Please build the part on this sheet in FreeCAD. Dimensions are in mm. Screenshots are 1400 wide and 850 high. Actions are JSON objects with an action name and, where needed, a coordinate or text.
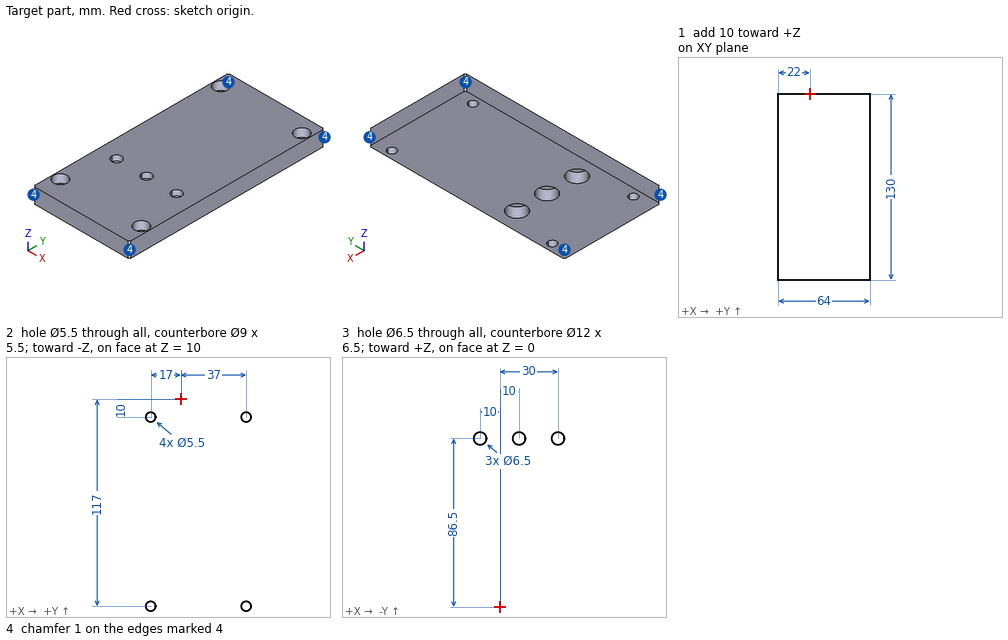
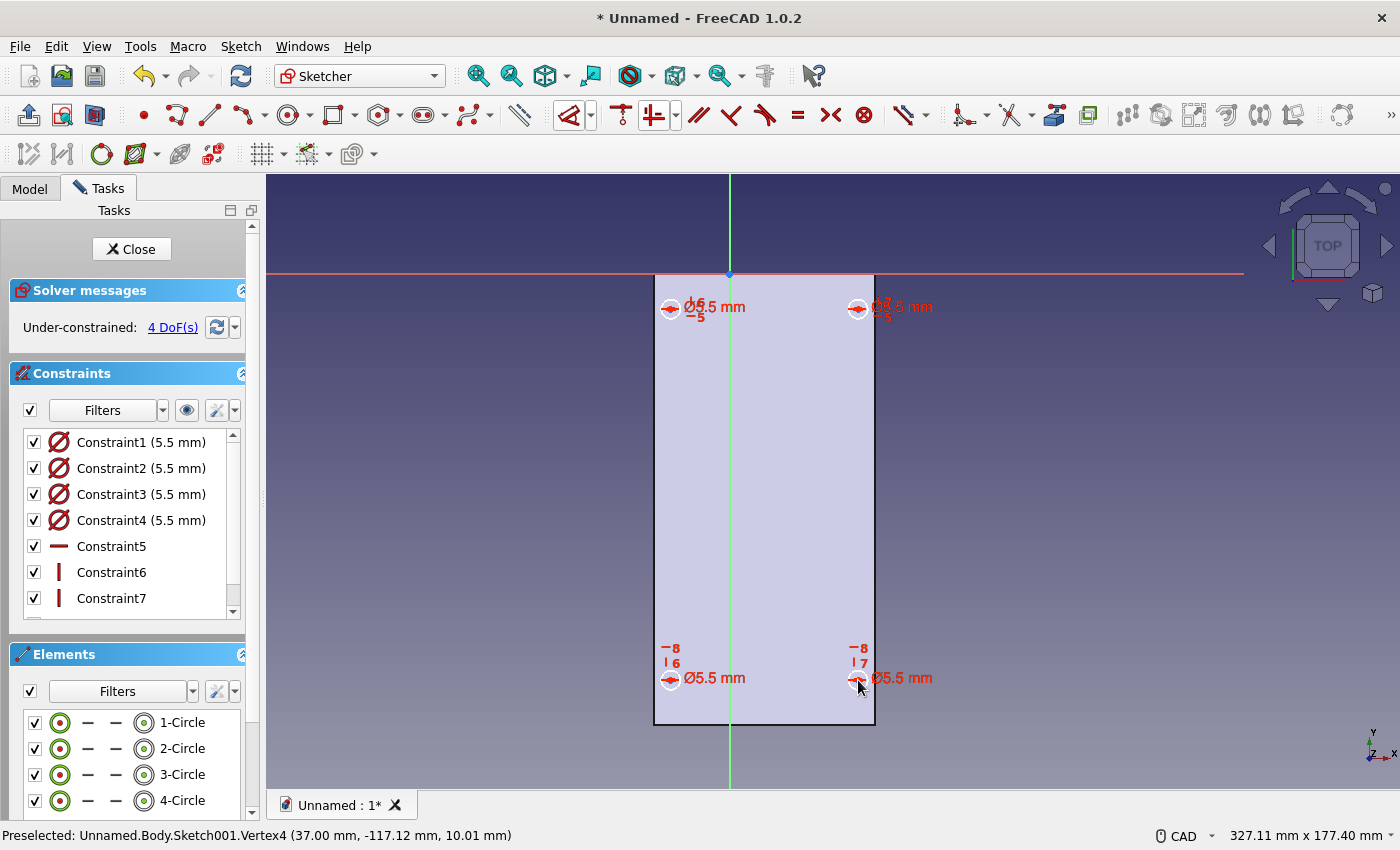
{"action": "left_click", "coordinate": [671, 309]}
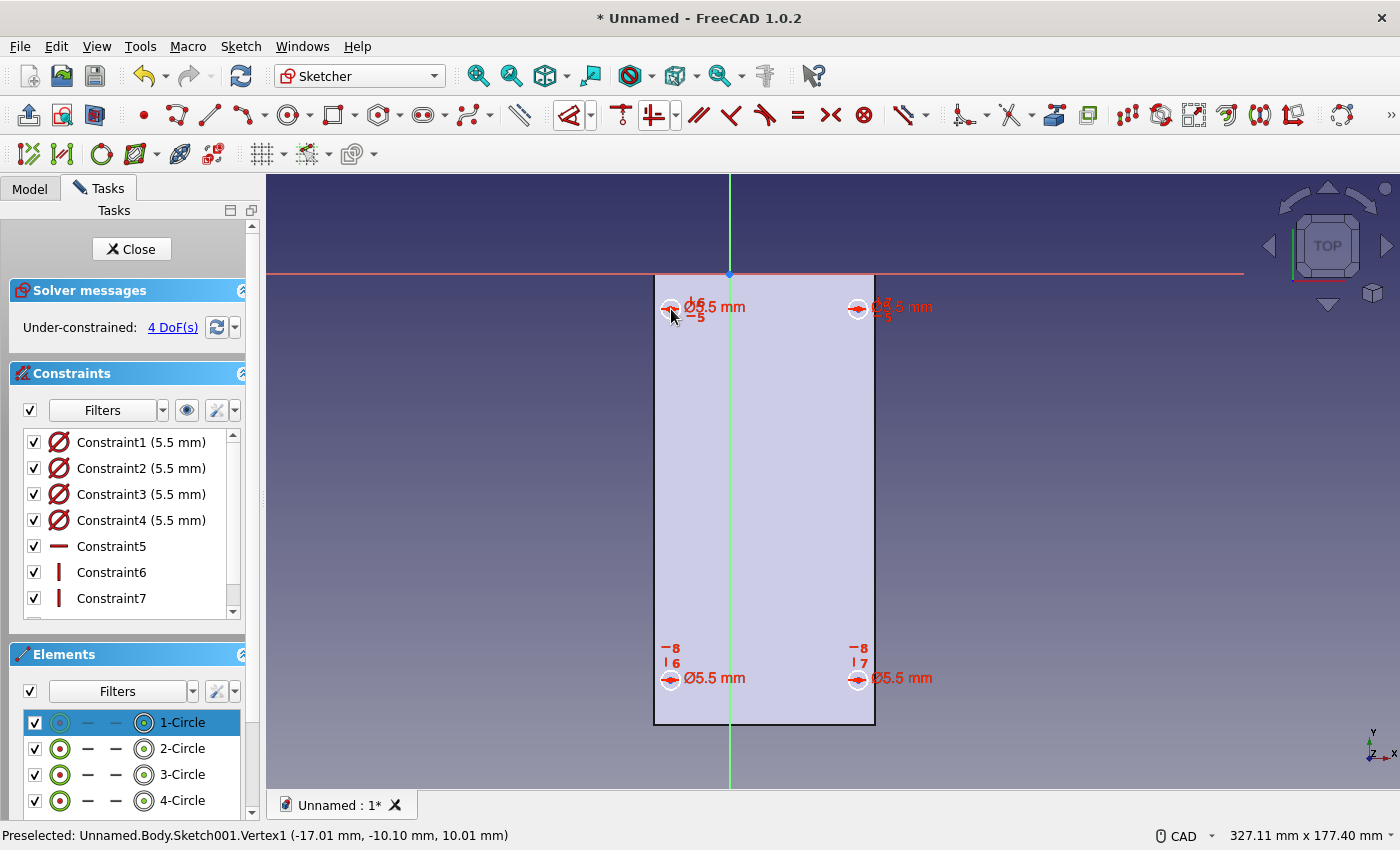
{"action": "key", "text": "l"}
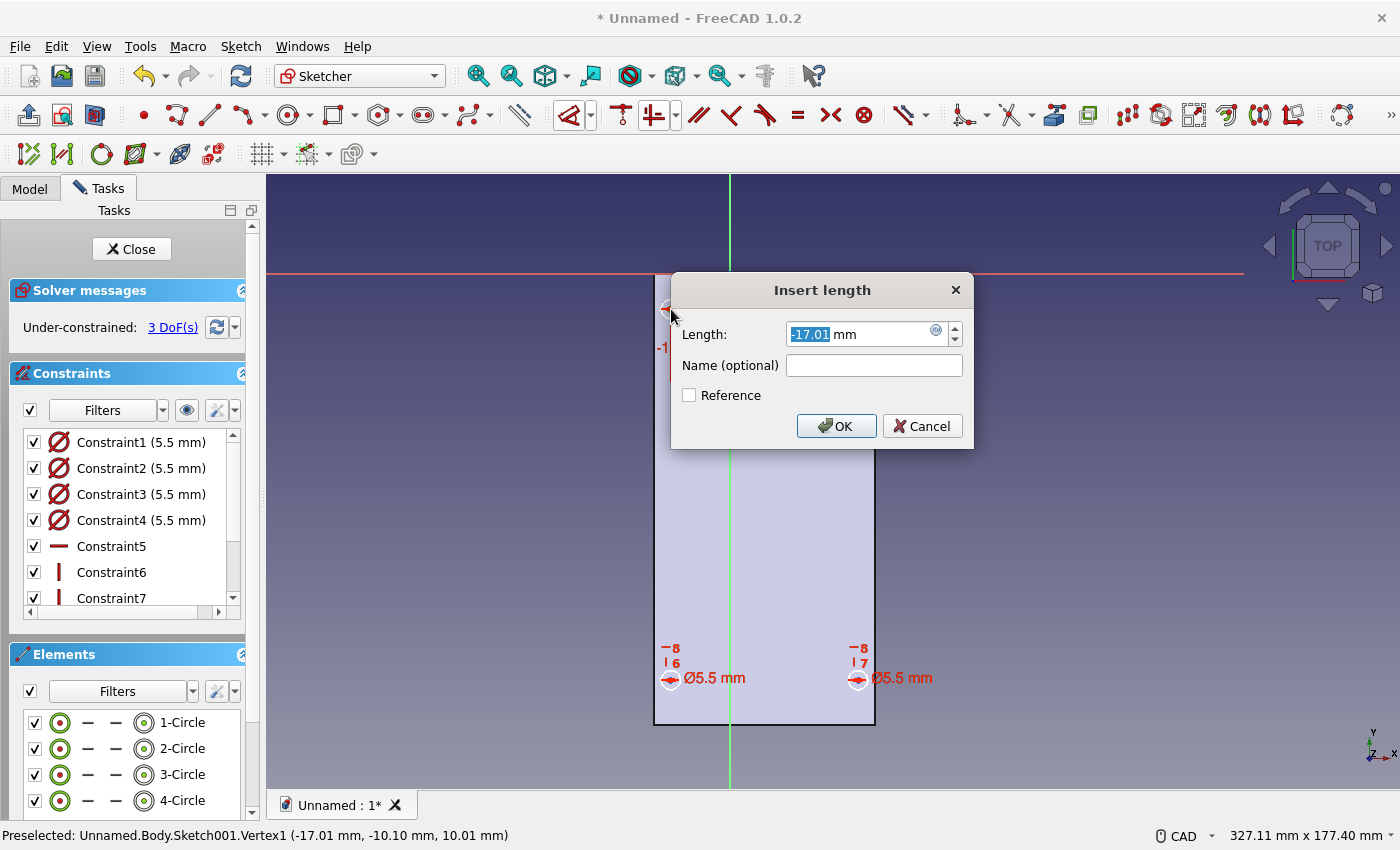
{"action": "type", "text": "-17"}
{"action": "key", "text": "Return"}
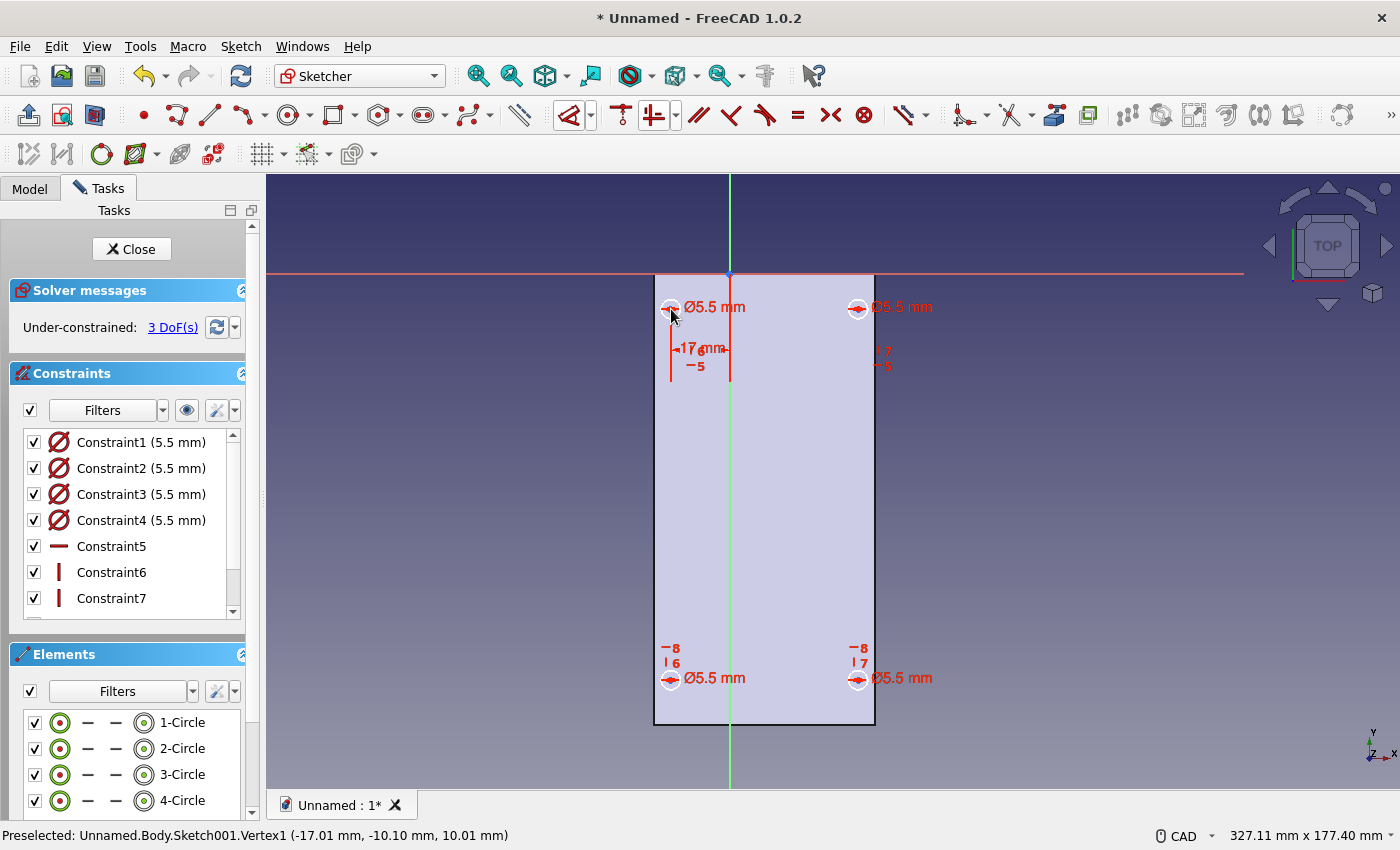
{"action": "left_click", "coordinate": [671, 309]}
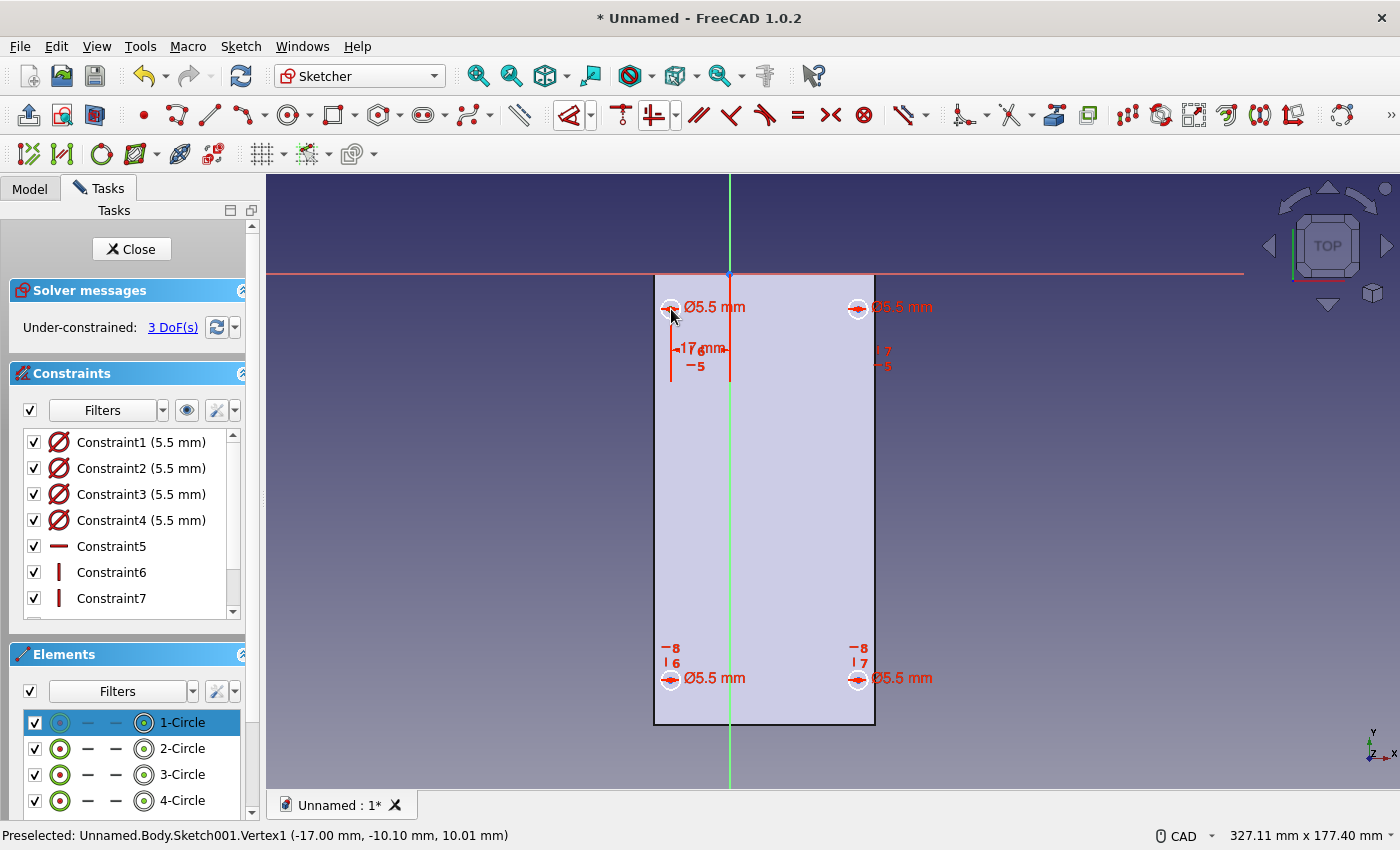
{"action": "key", "text": "i"}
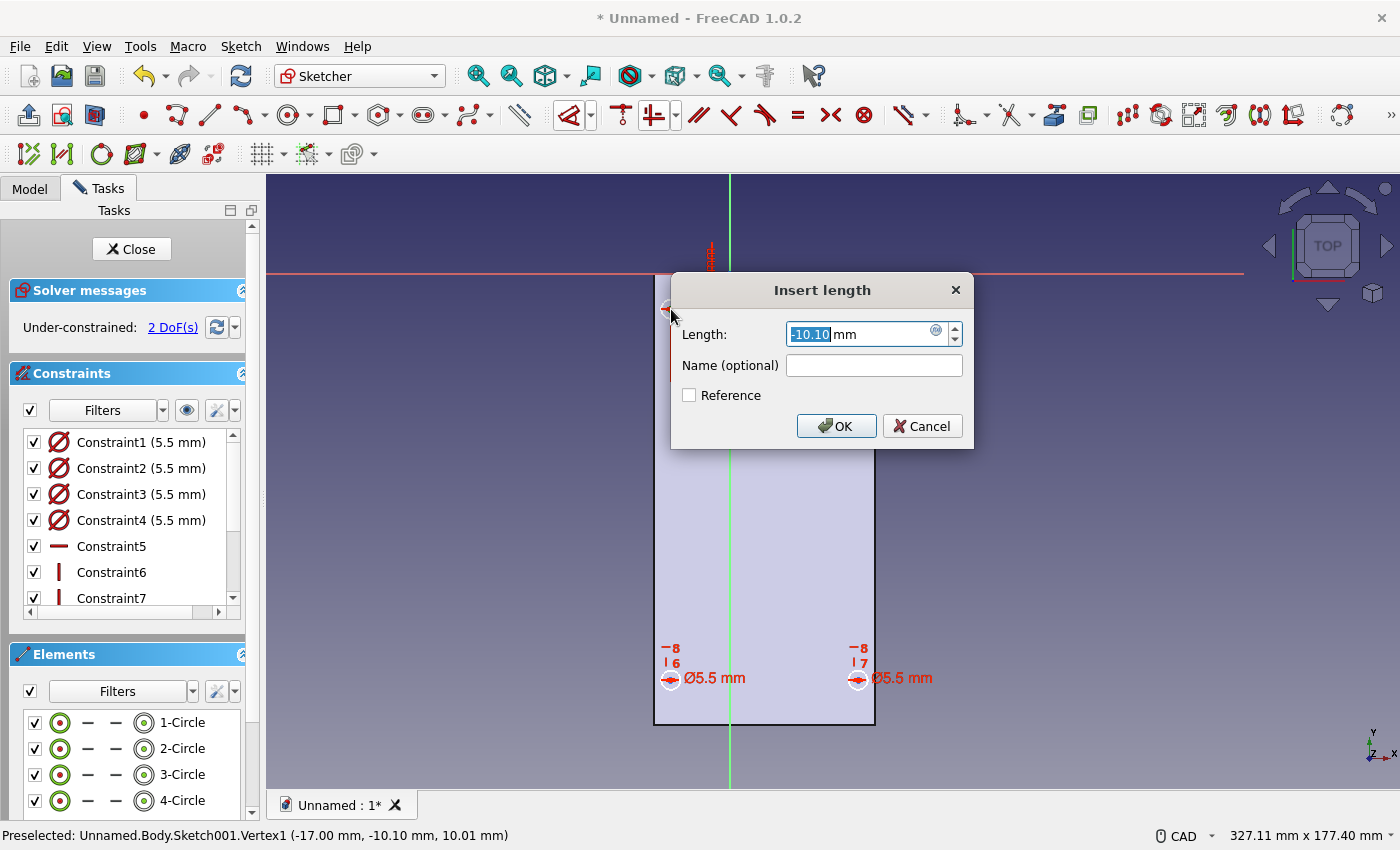
{"action": "type", "text": "-10"}
{"action": "key", "text": "Return"}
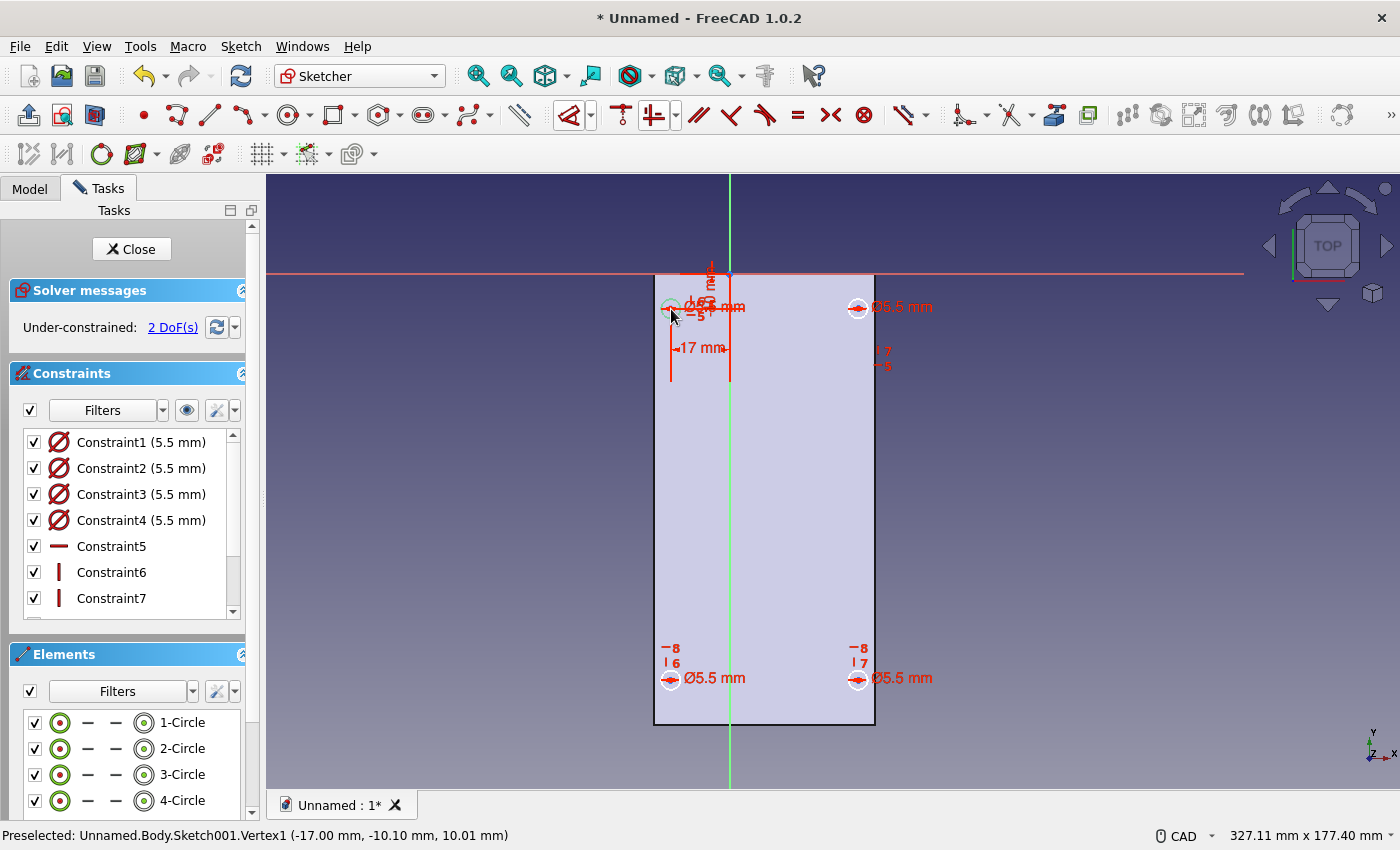
{"action": "left_click", "coordinate": [858, 309]}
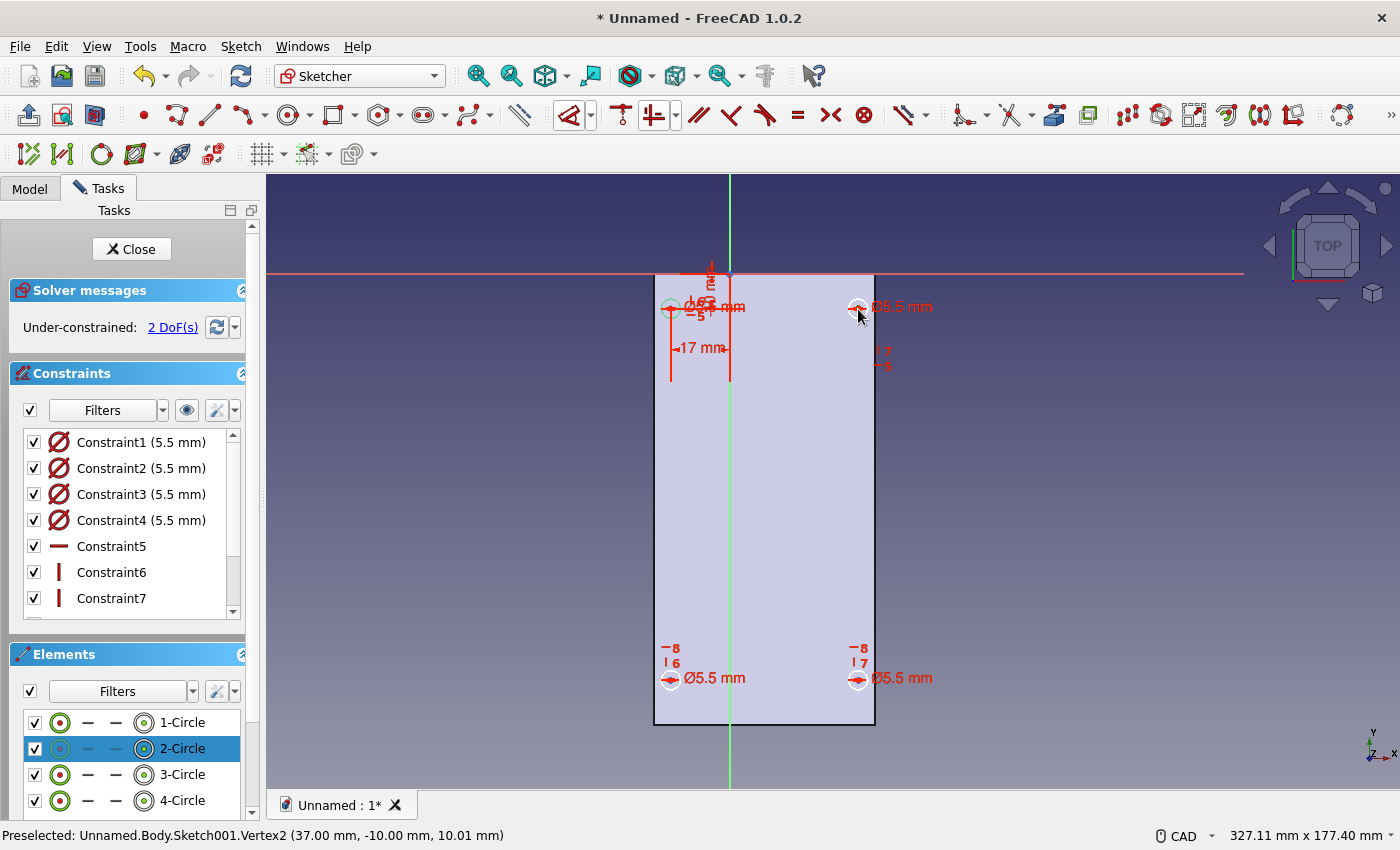
{"action": "key", "text": "l"}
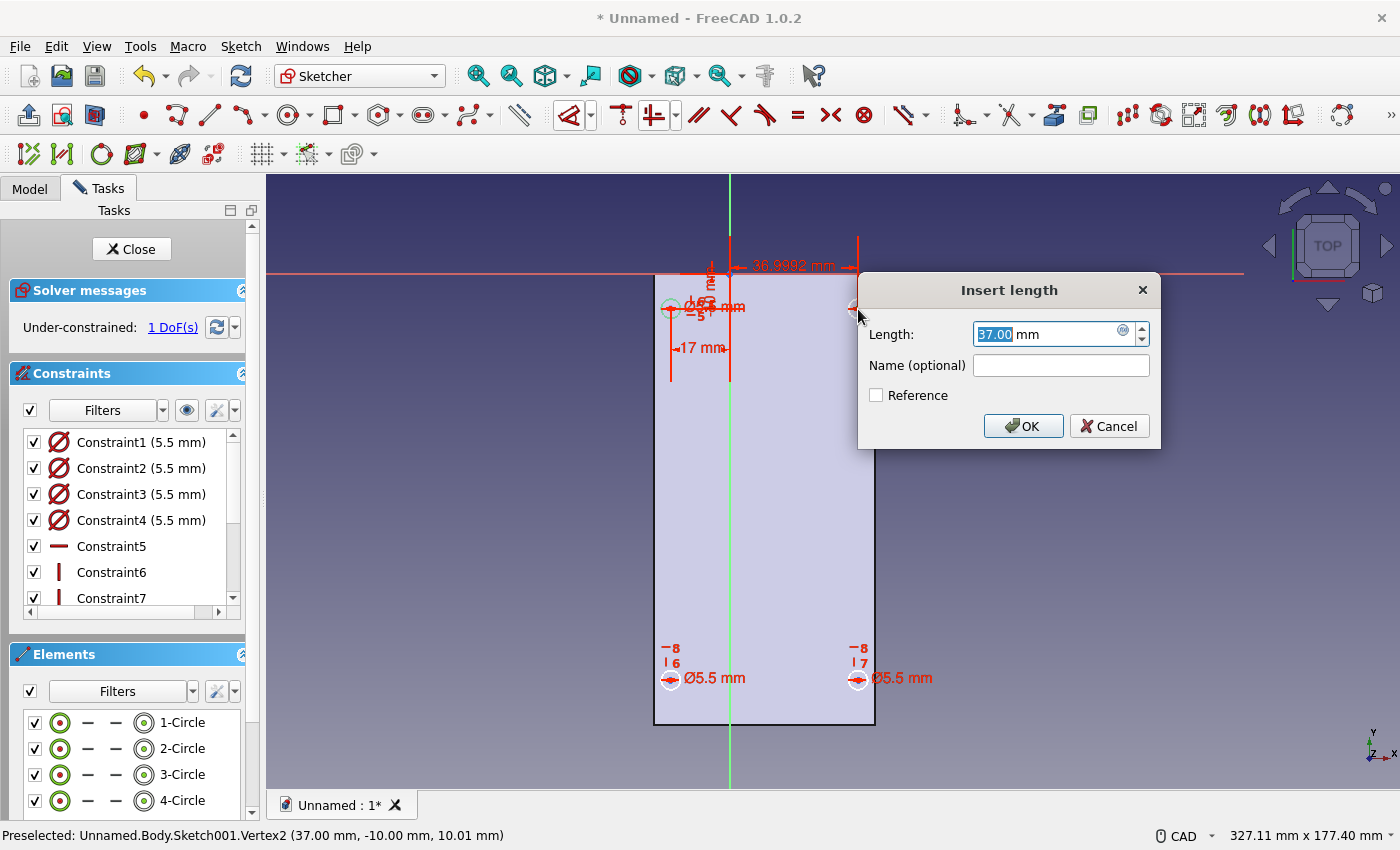
{"action": "type", "text": "37"}
{"action": "key", "text": "Return"}